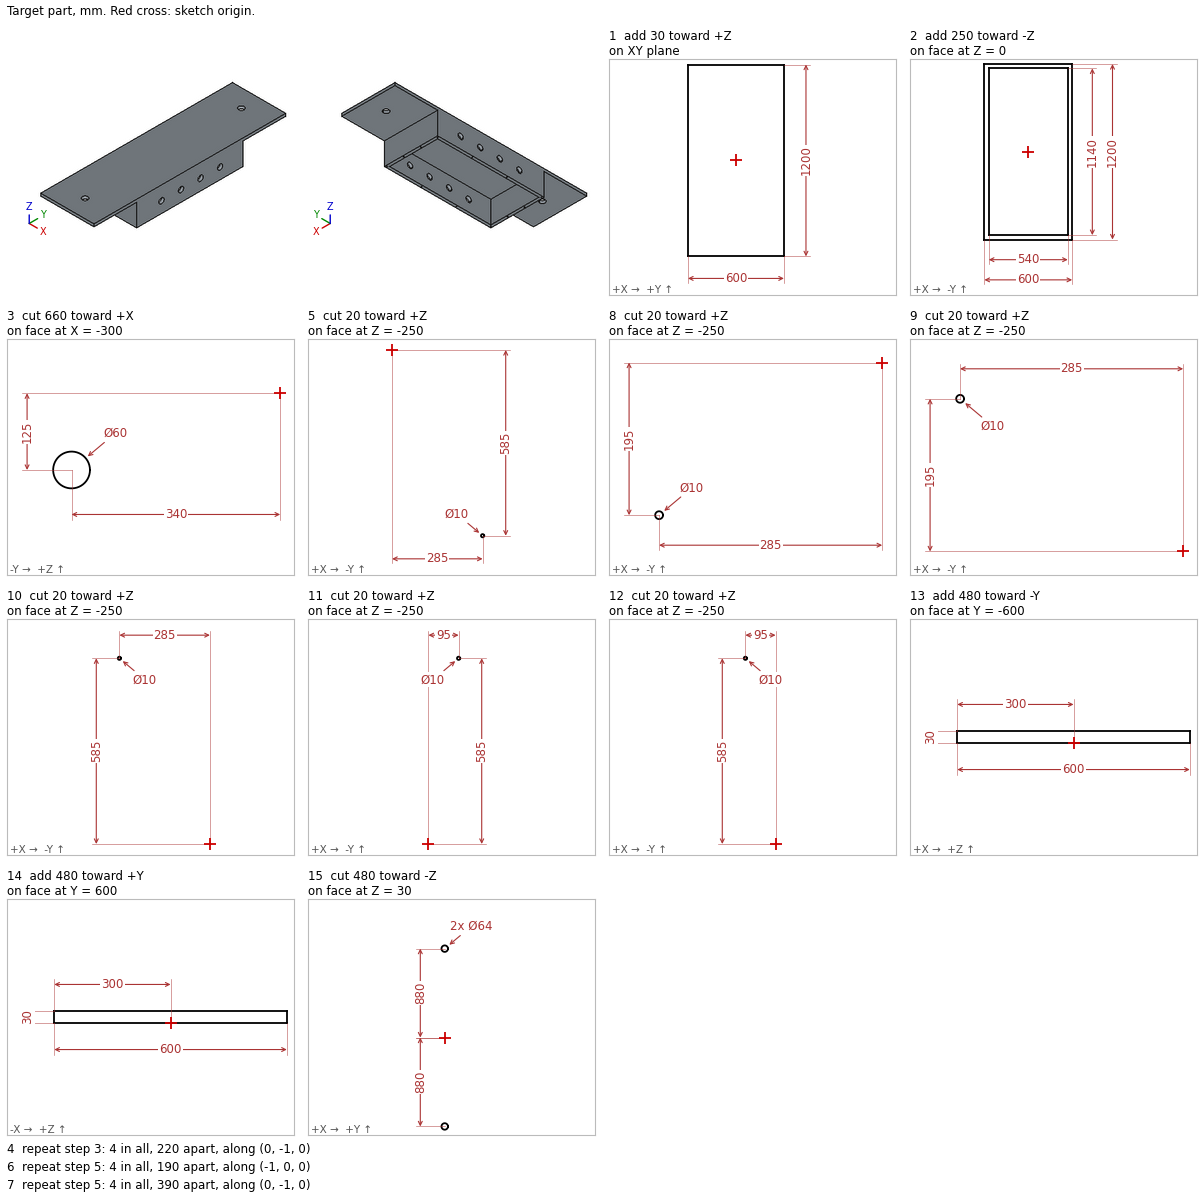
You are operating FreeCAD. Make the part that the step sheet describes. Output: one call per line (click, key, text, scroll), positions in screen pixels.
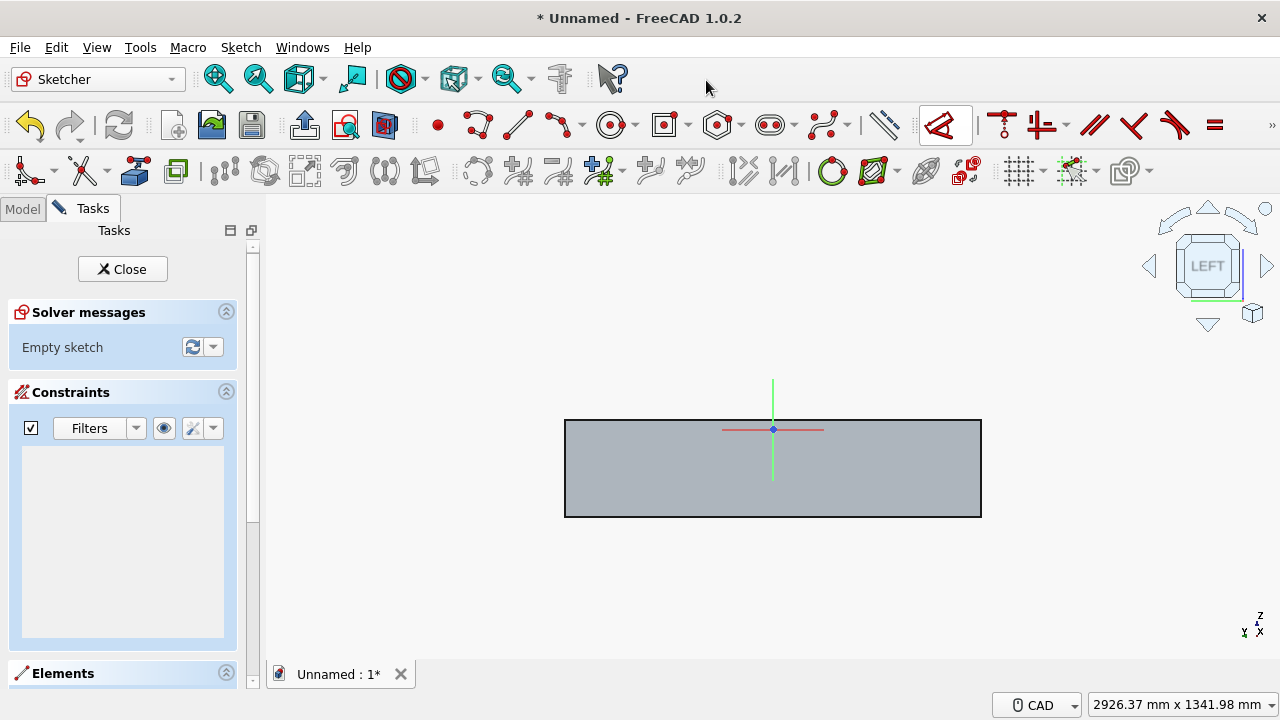
scroll(651, 477, up, 13)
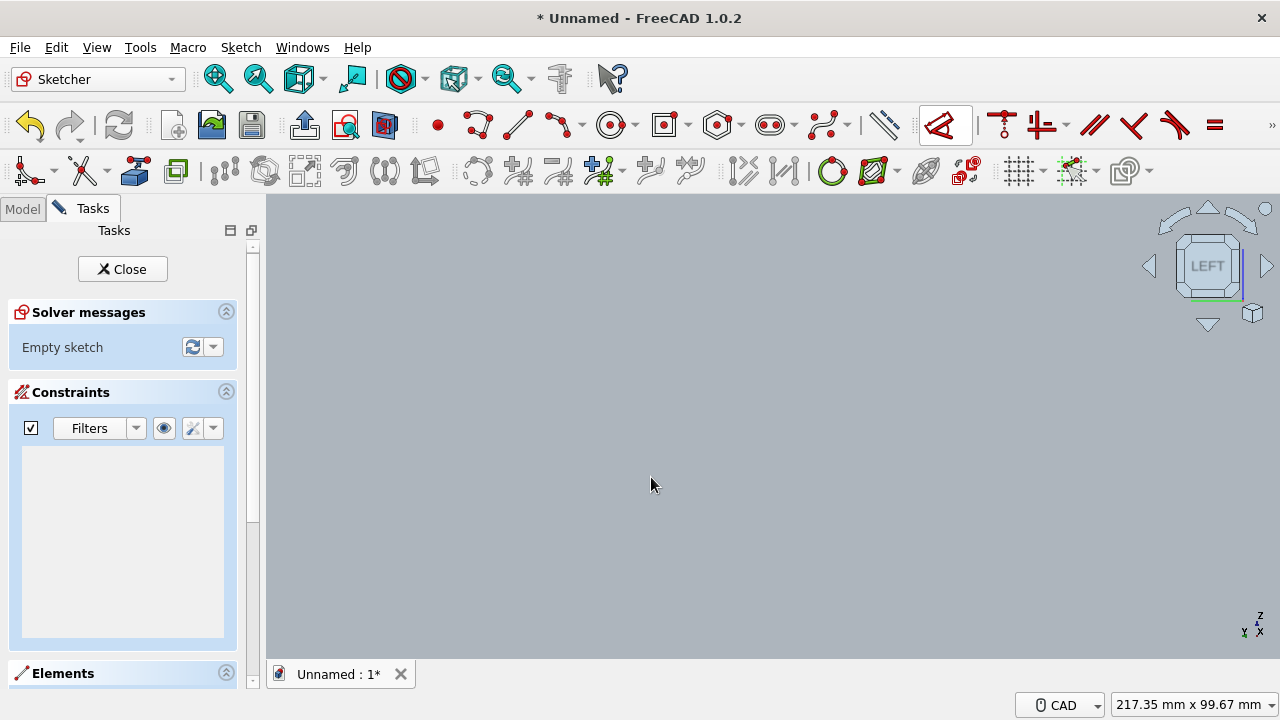
click(612, 126)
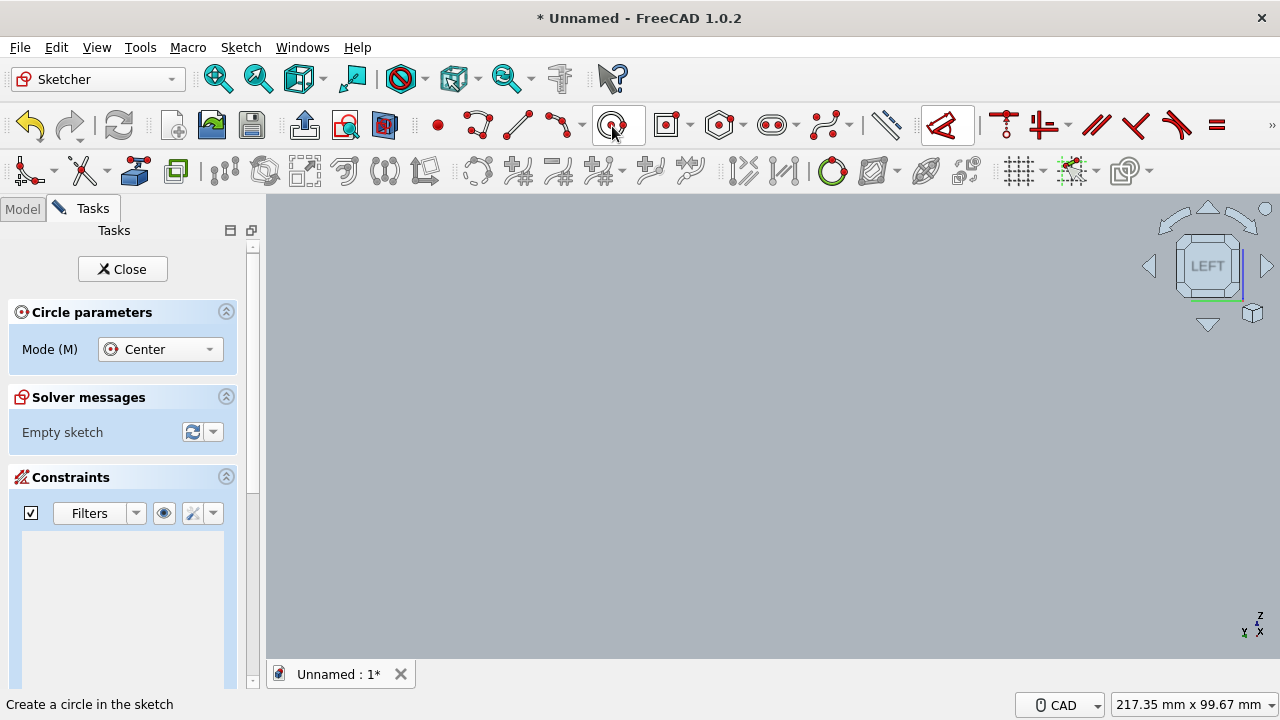
click(703, 419)
move(802, 320)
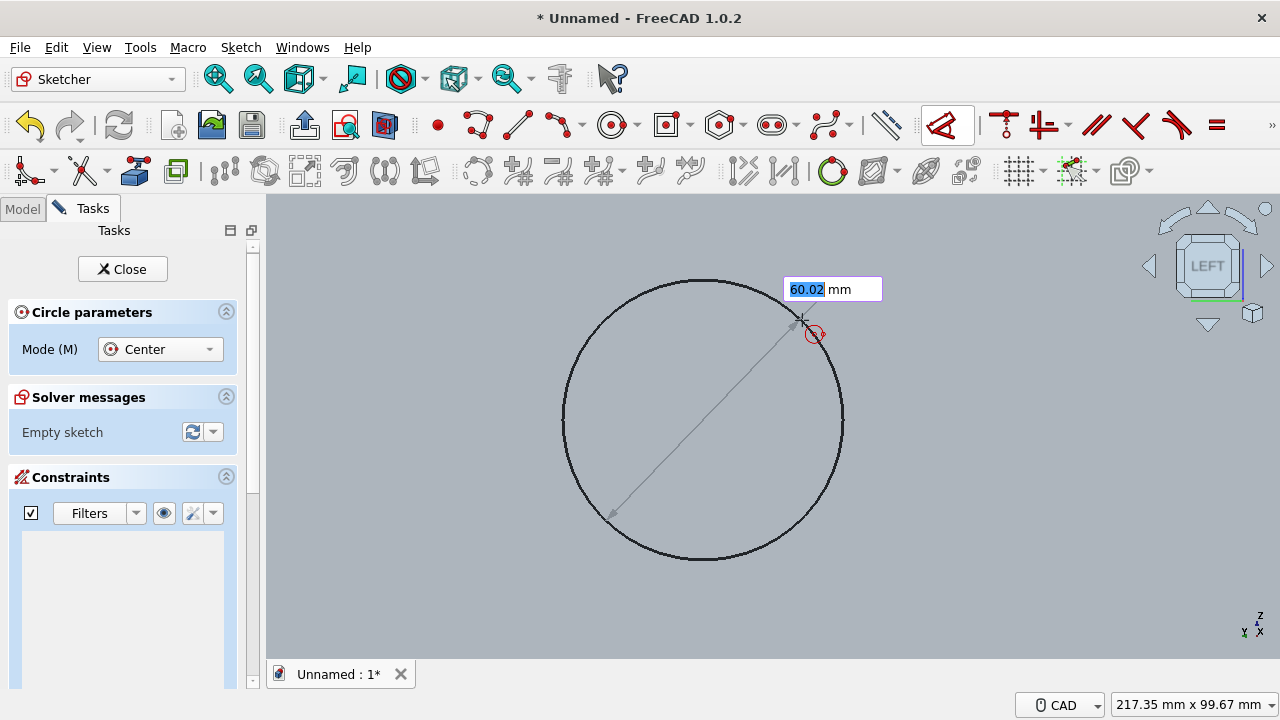
text(60)
key(Return)
key(Escape)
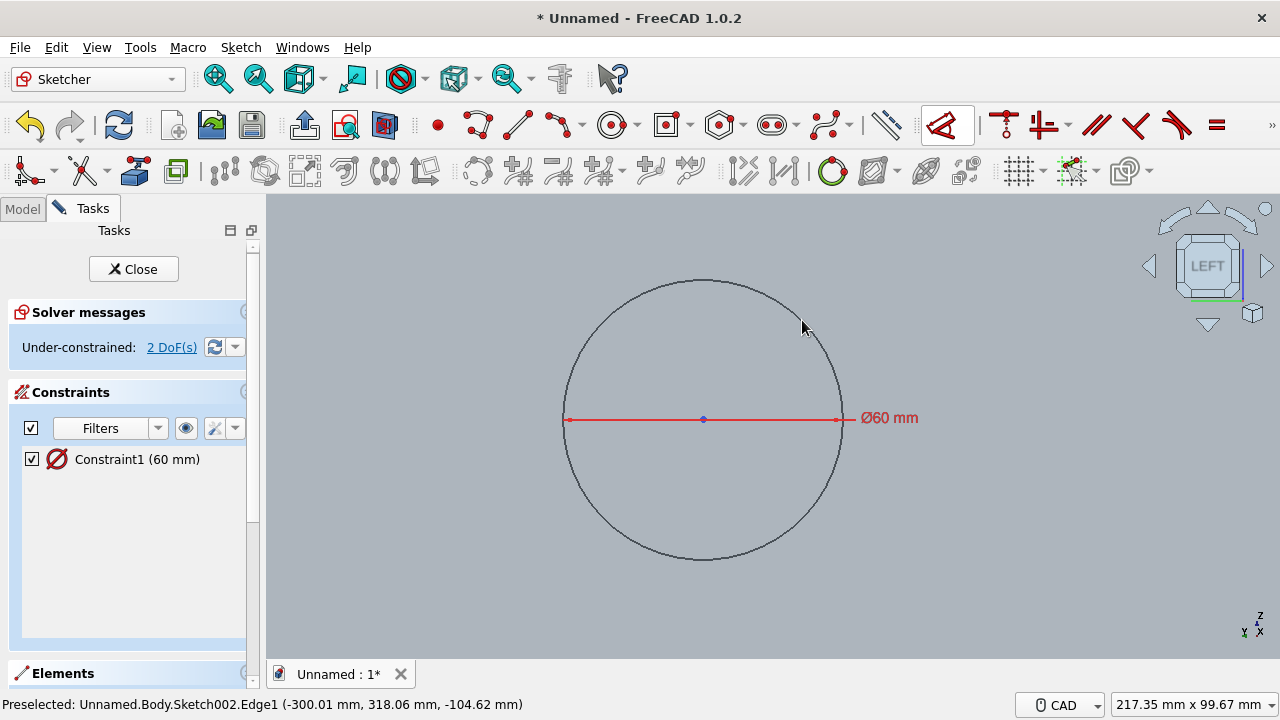
click(703, 420)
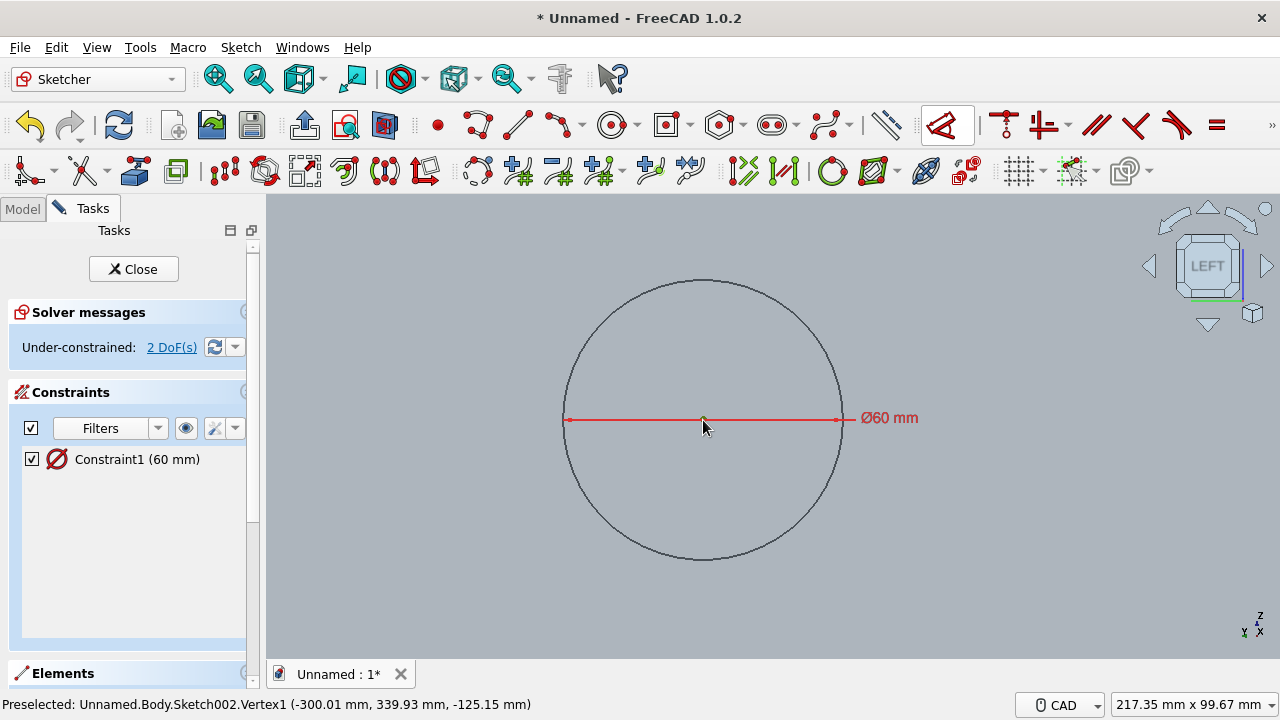
click(968, 126)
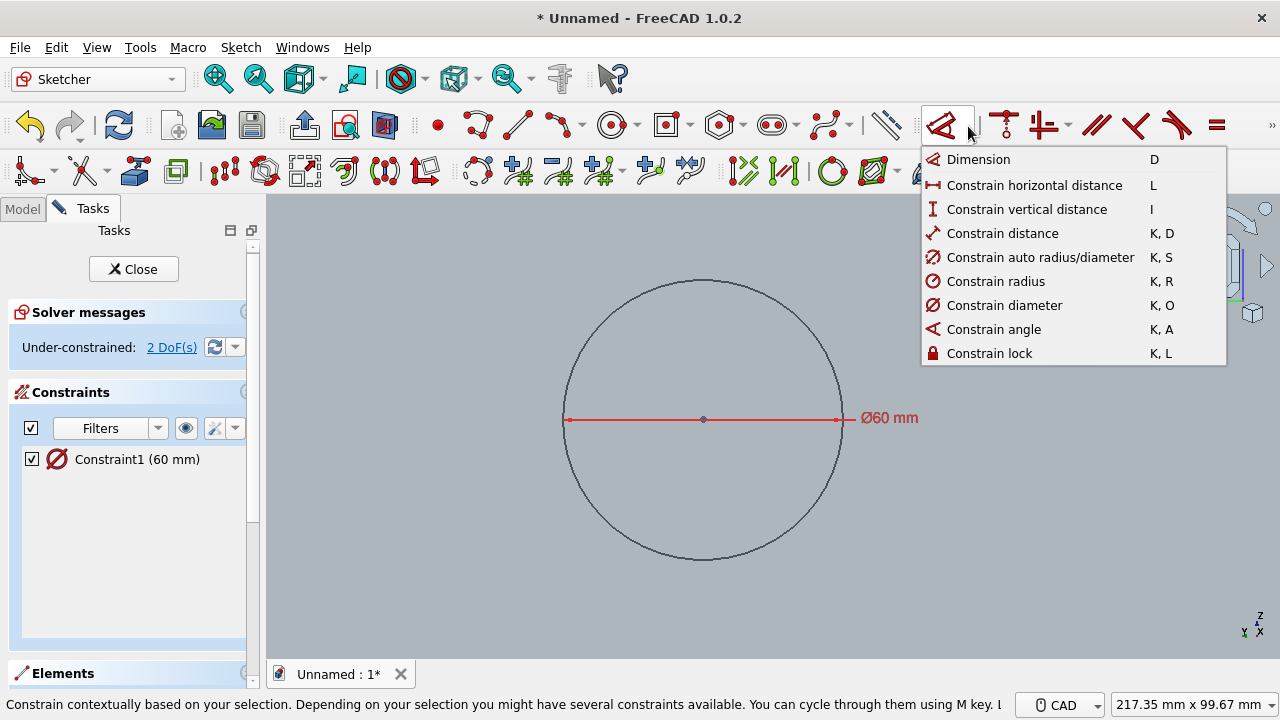
click(1074, 185)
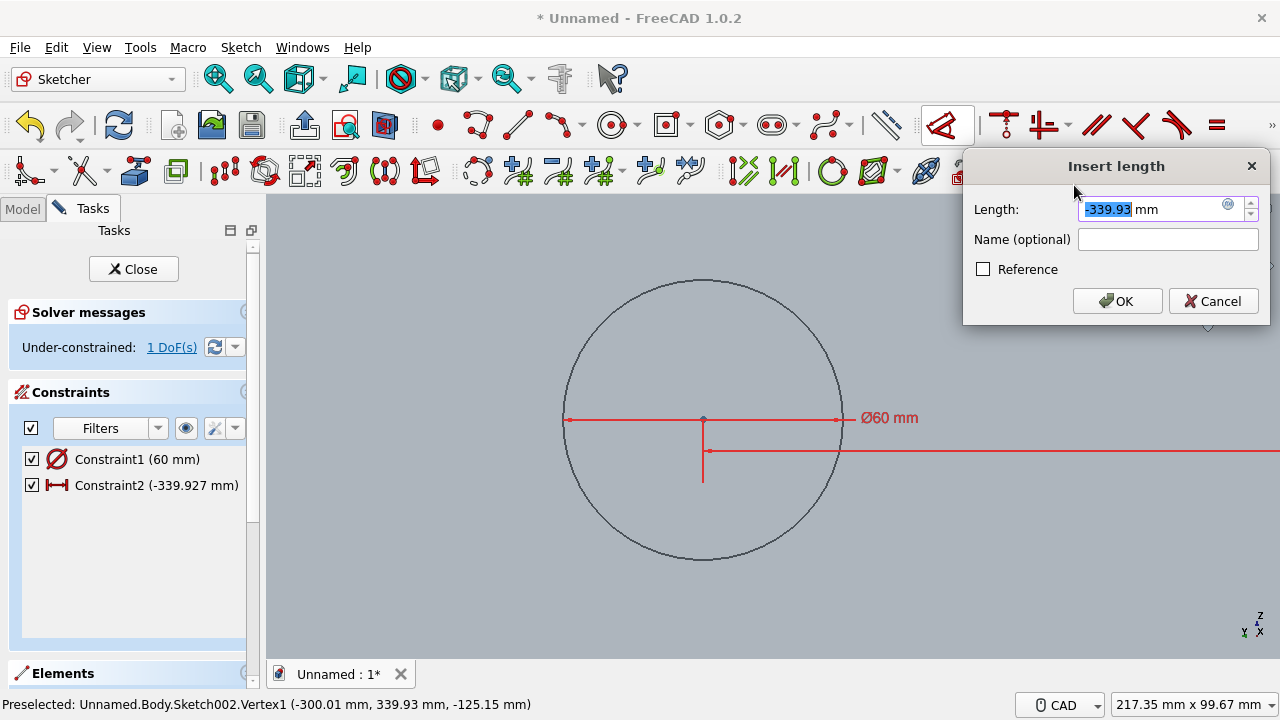
text(-340)
key(Return)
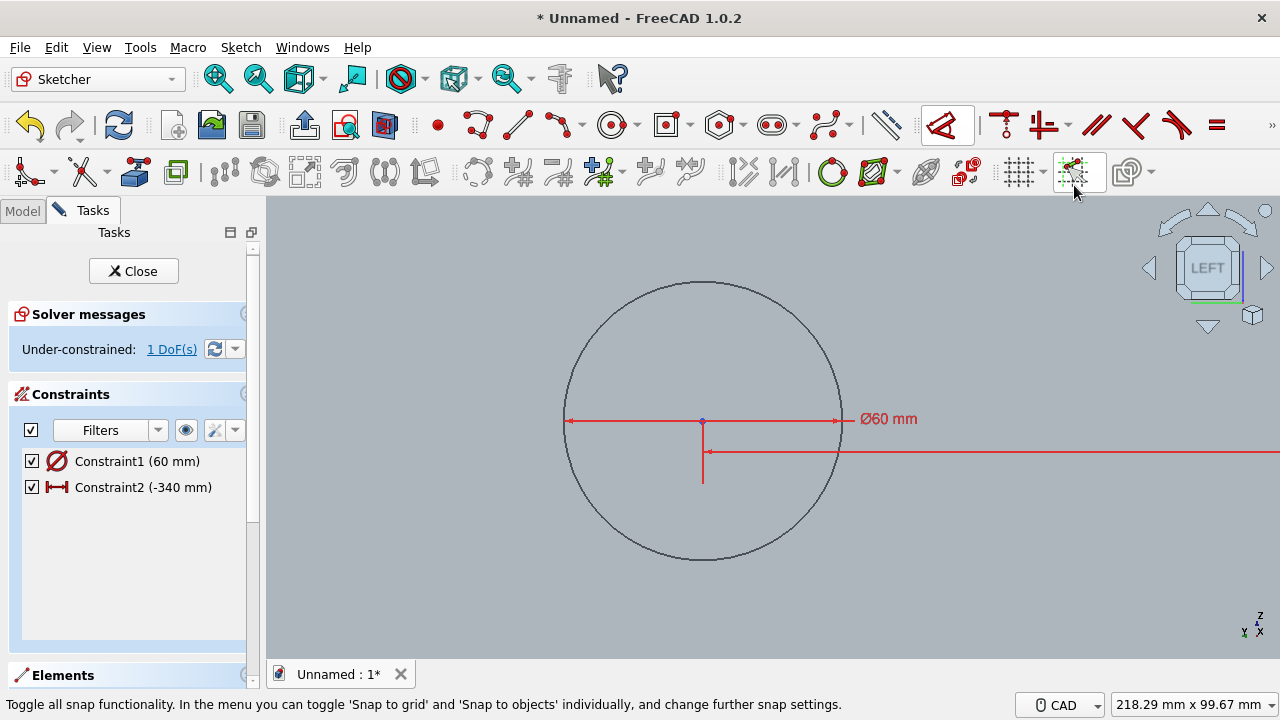
click(703, 421)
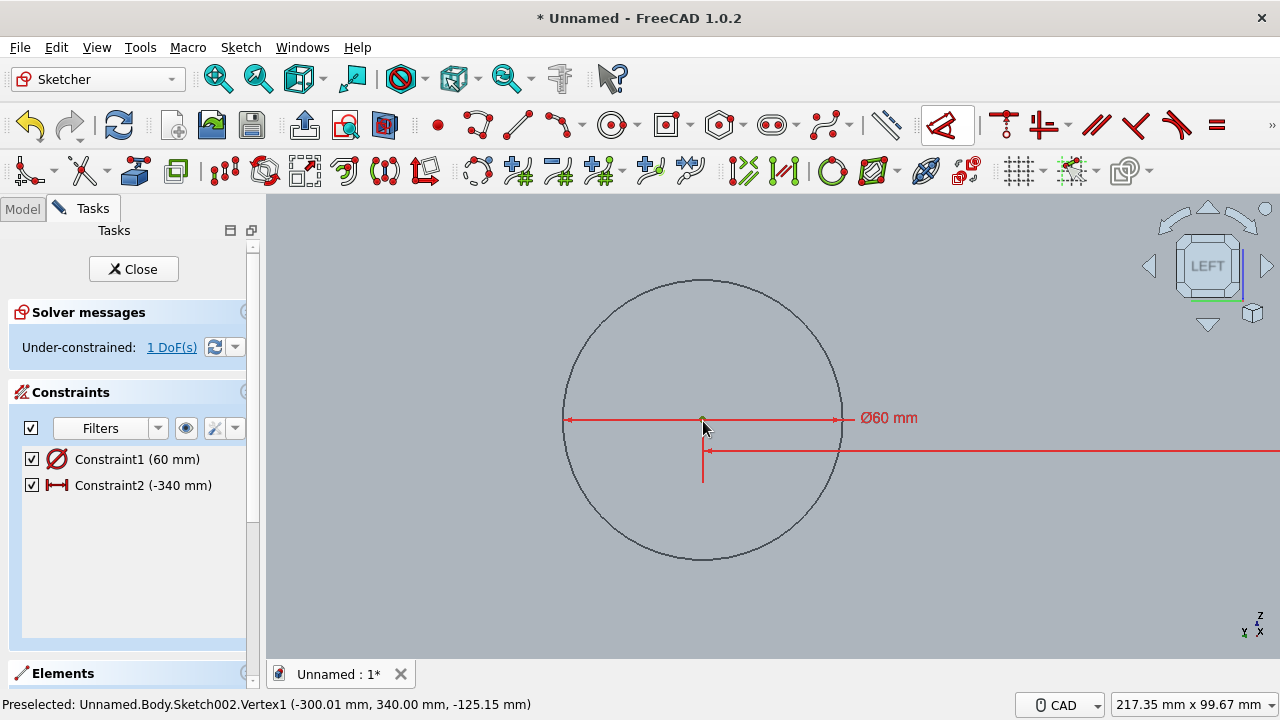
key(i)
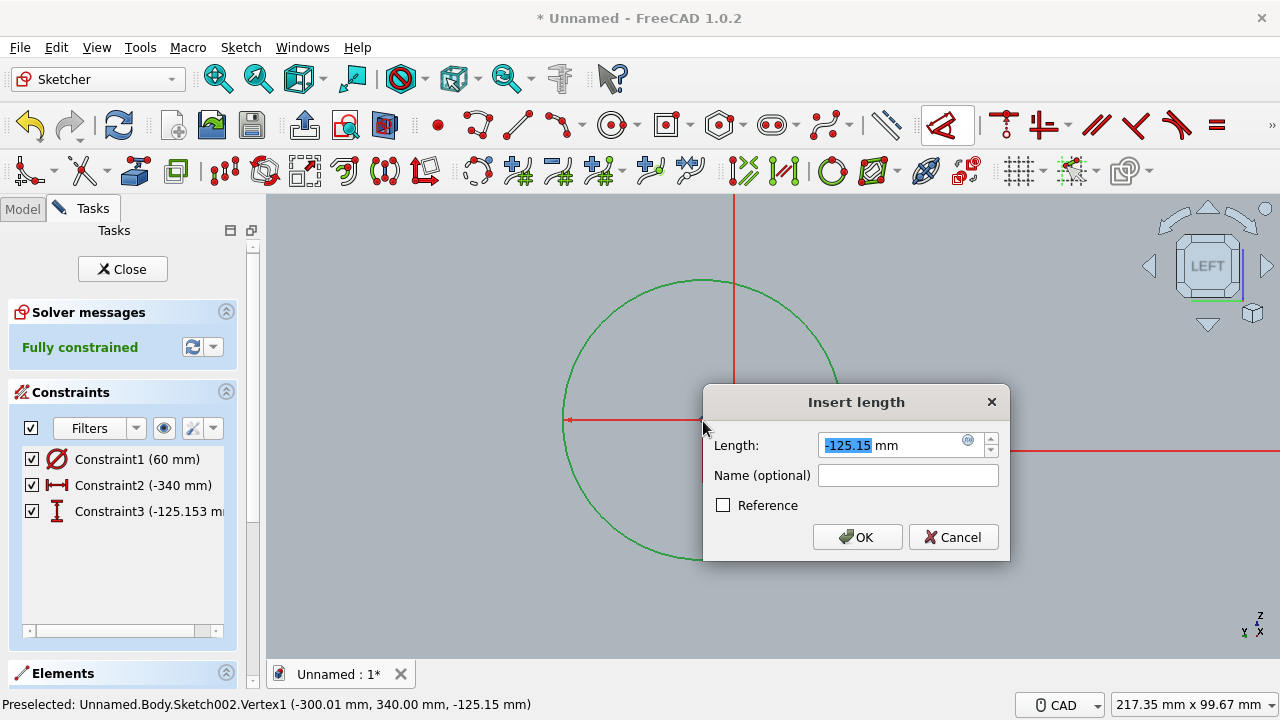
text(-125)
key(Return)